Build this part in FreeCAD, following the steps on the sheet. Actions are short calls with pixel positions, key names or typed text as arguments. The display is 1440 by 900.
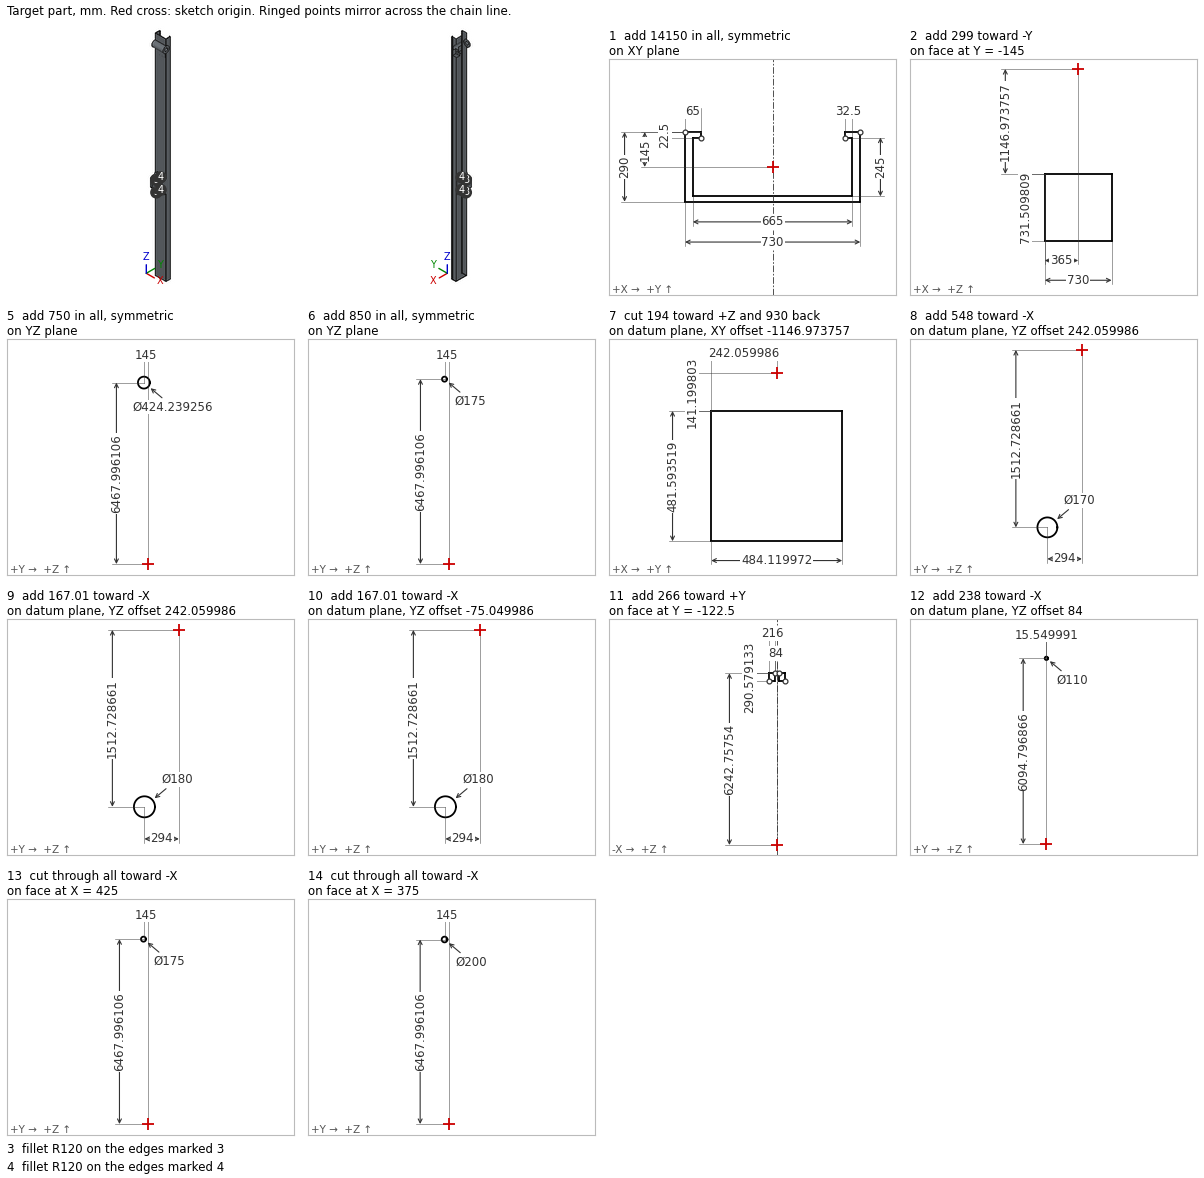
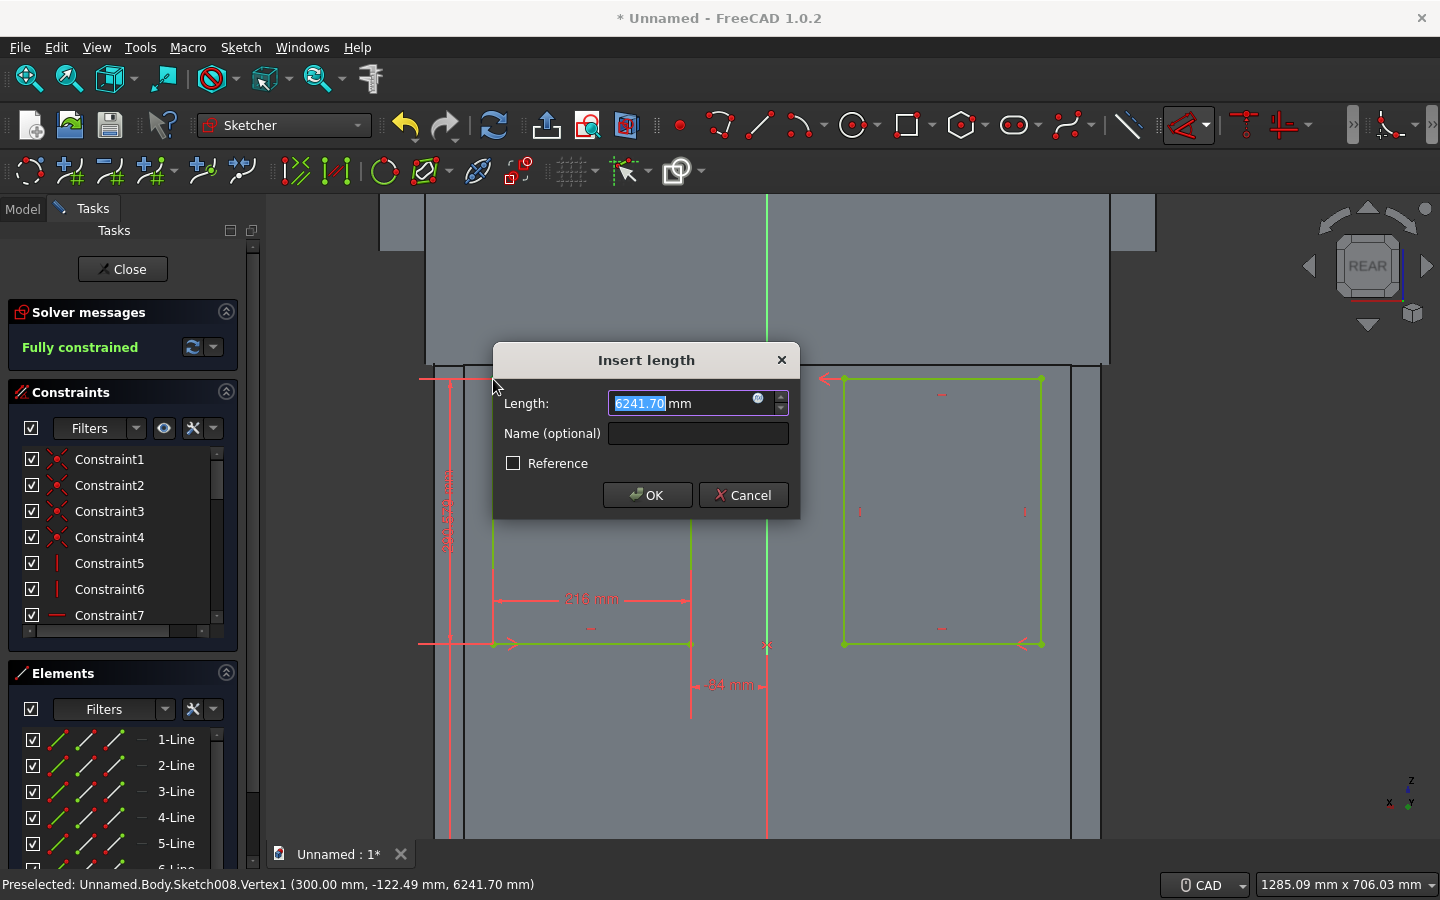
text(6242.75754)
key(Return)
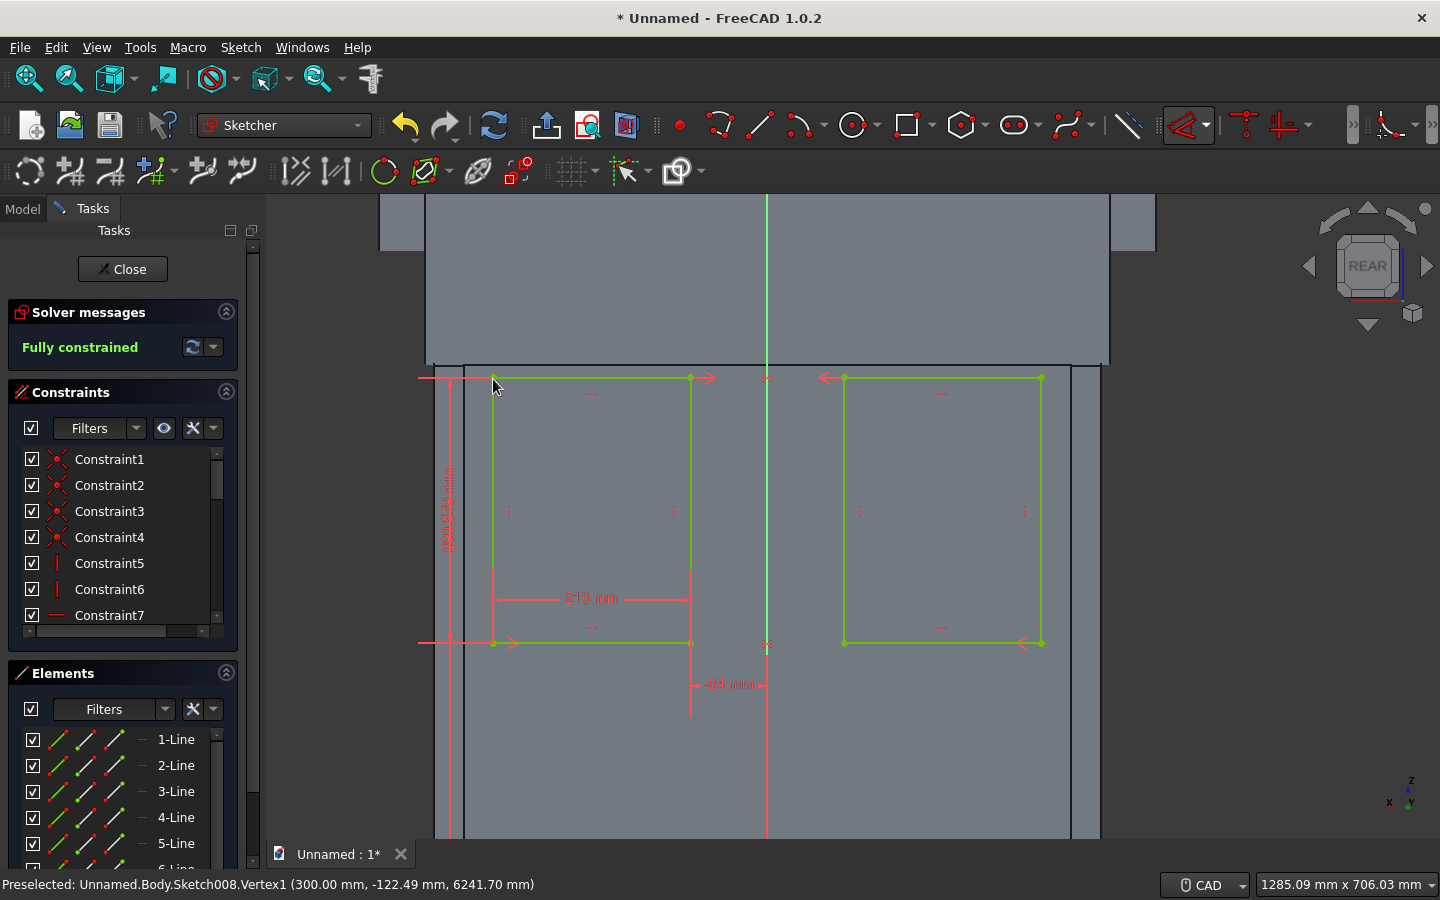
click(123, 269)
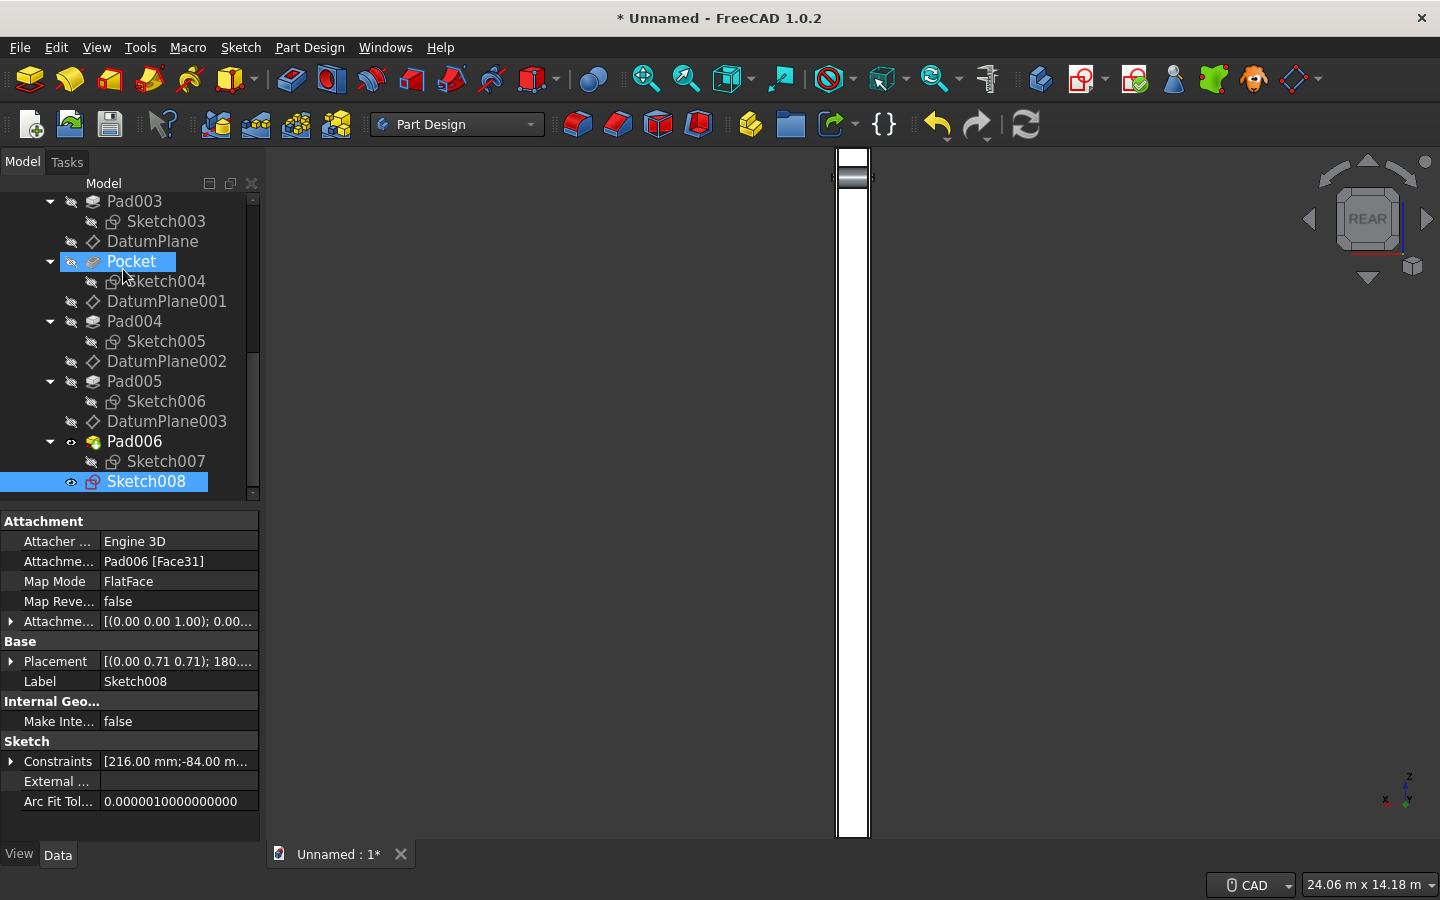
click(30, 80)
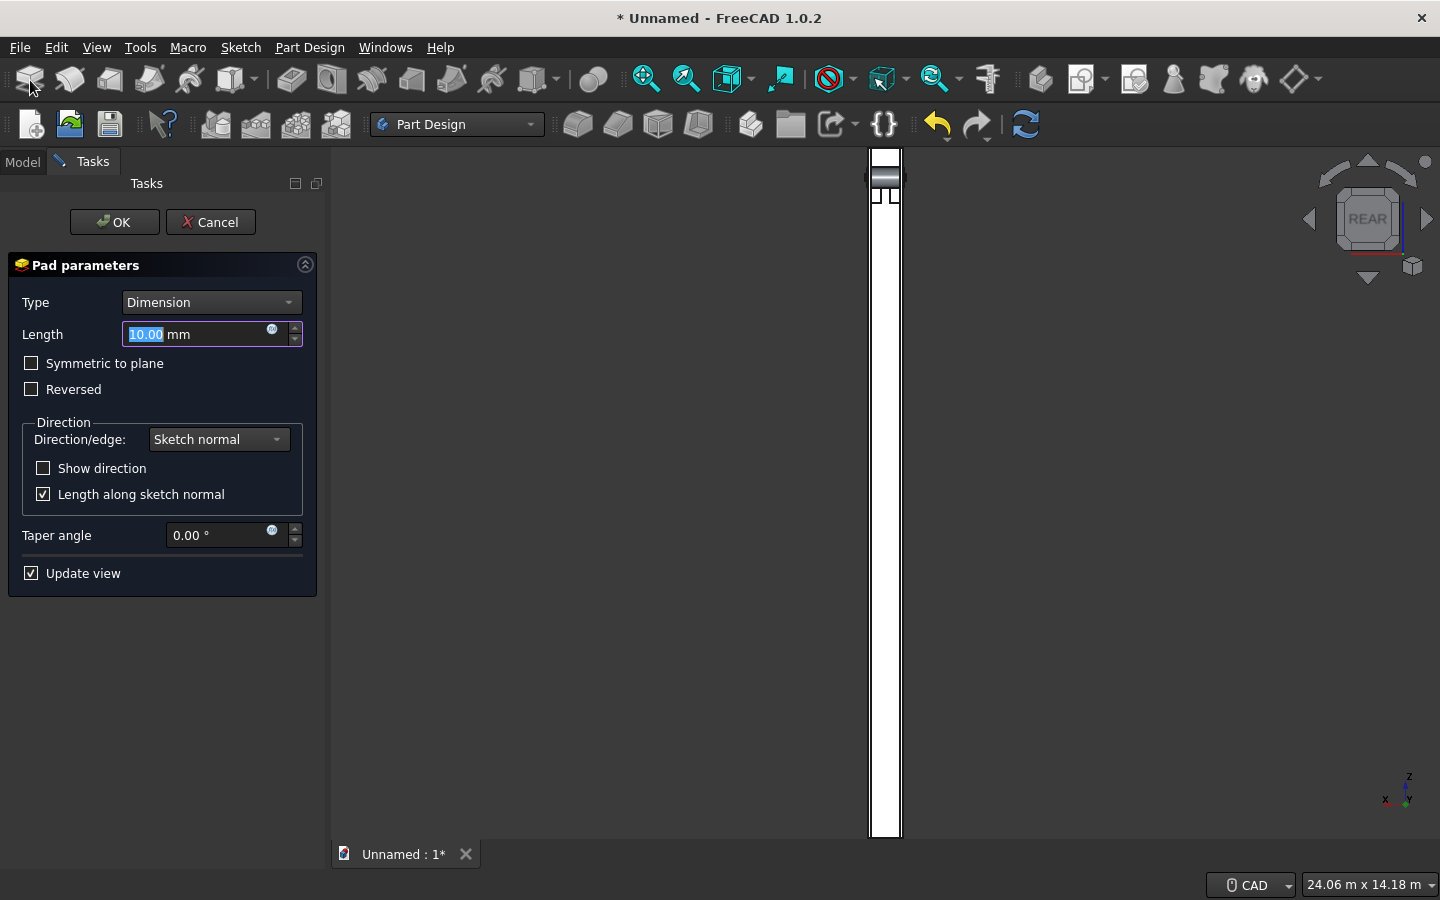
text(266)
key(Tab)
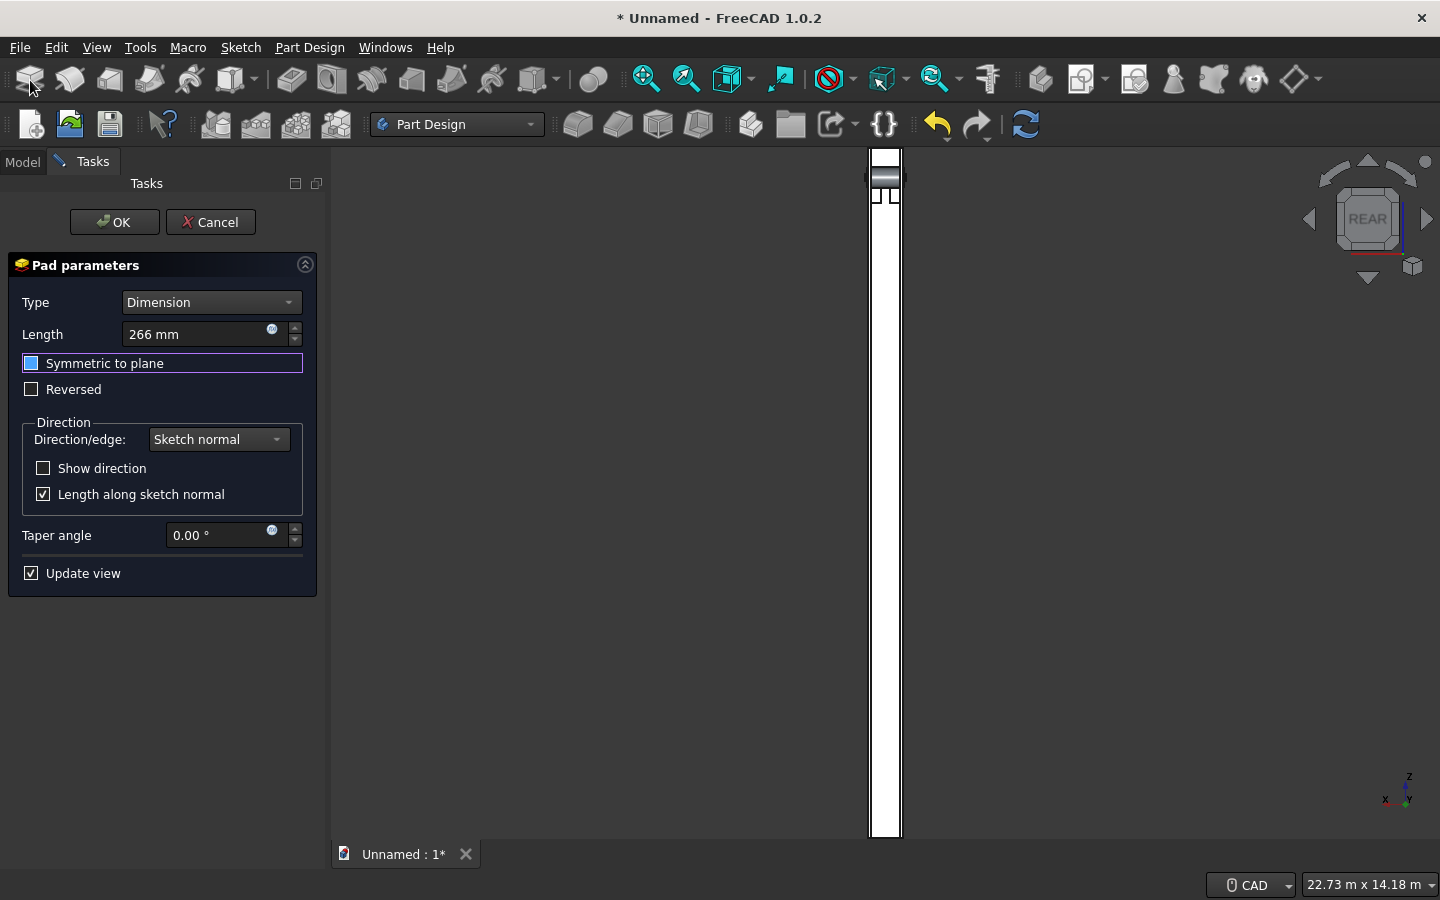
click(115, 222)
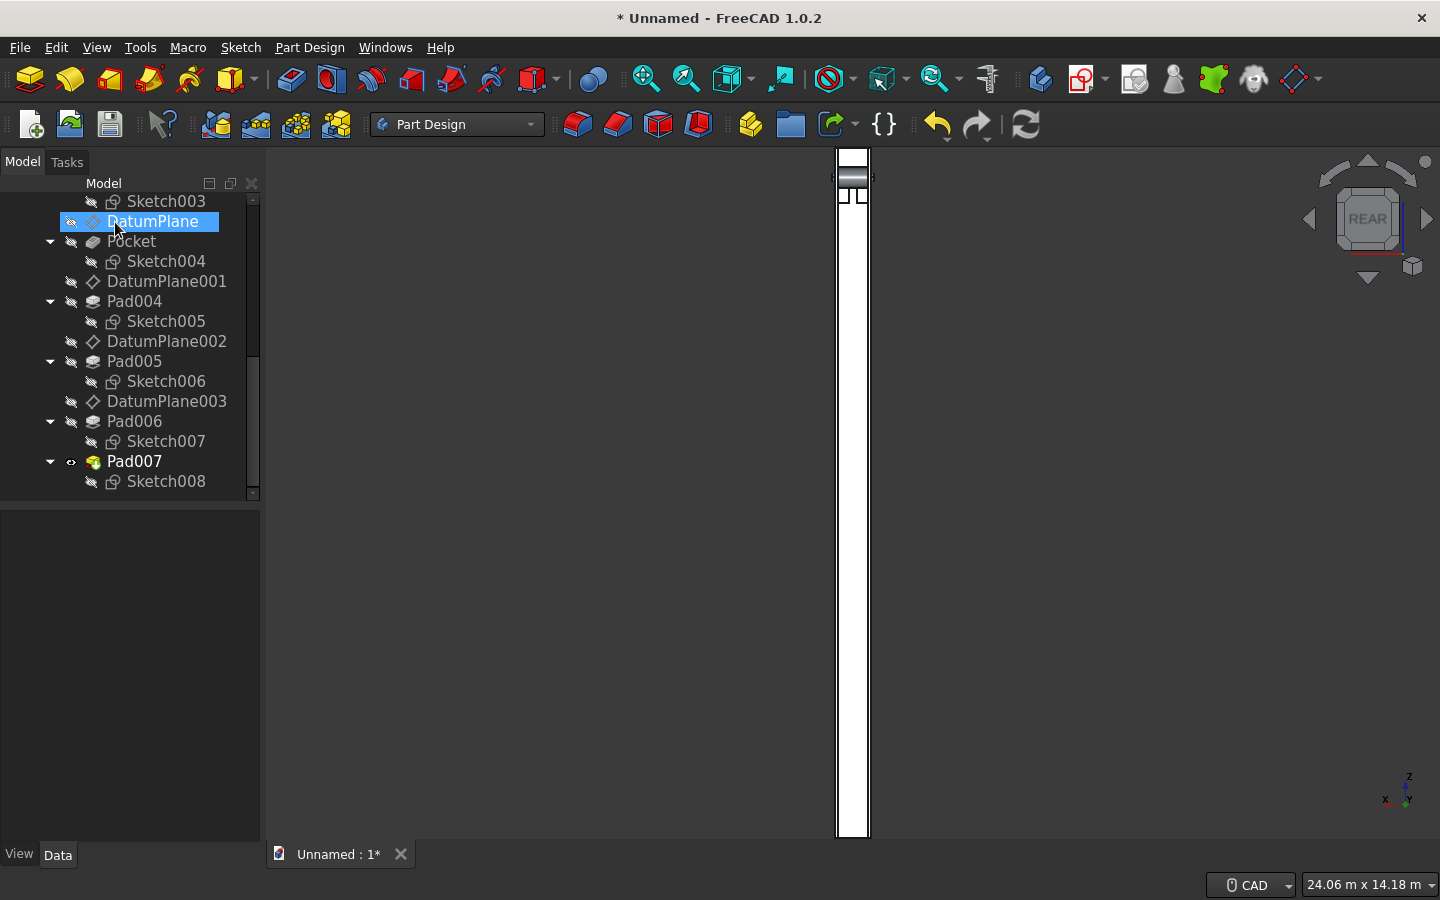
scroll(160, 337, down, 3)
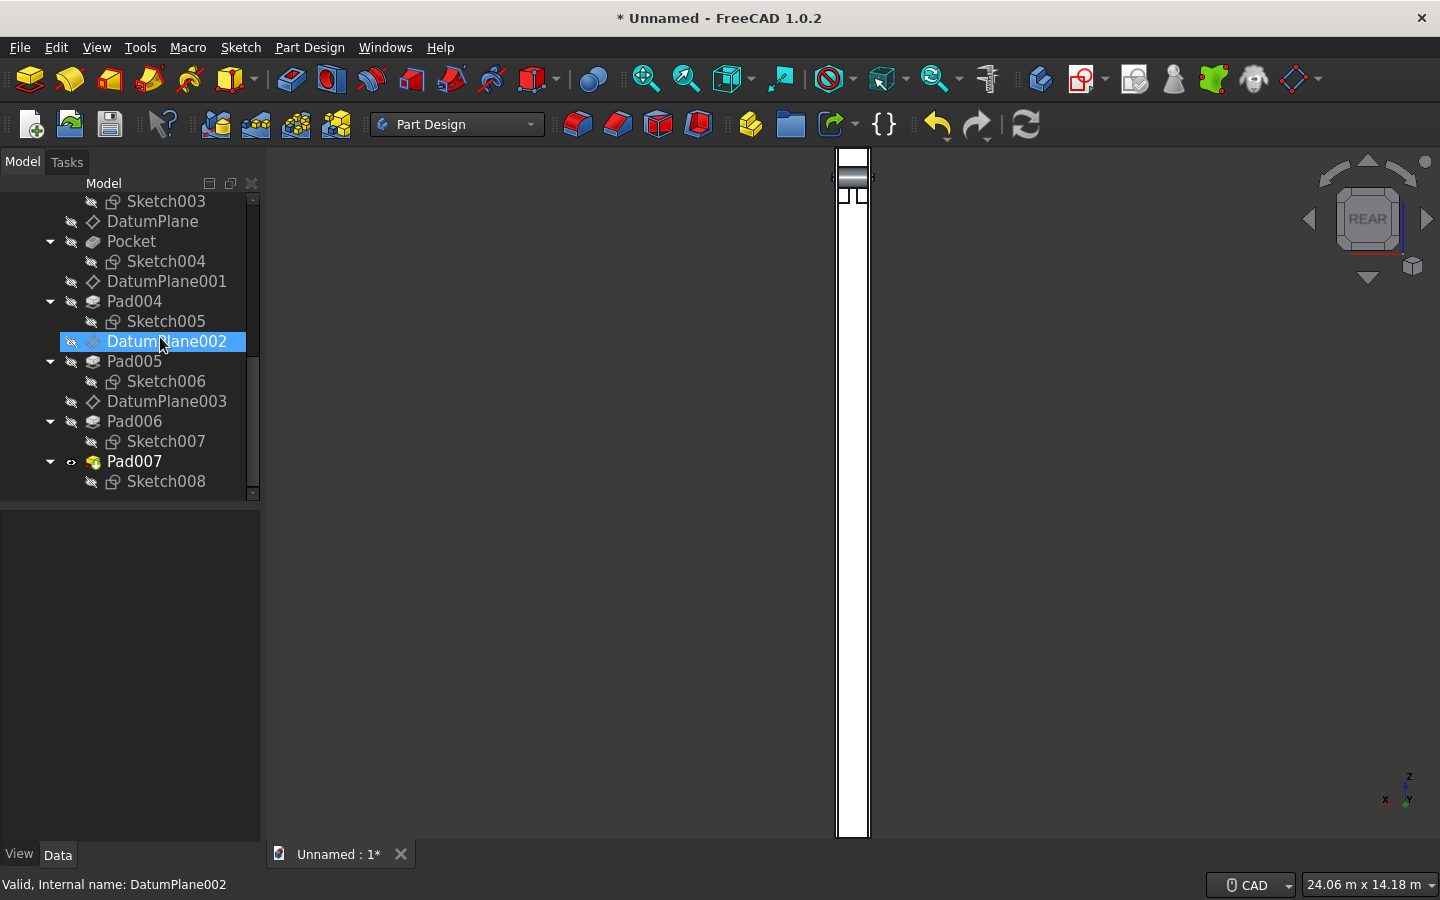
scroll(160, 337, up, 15)